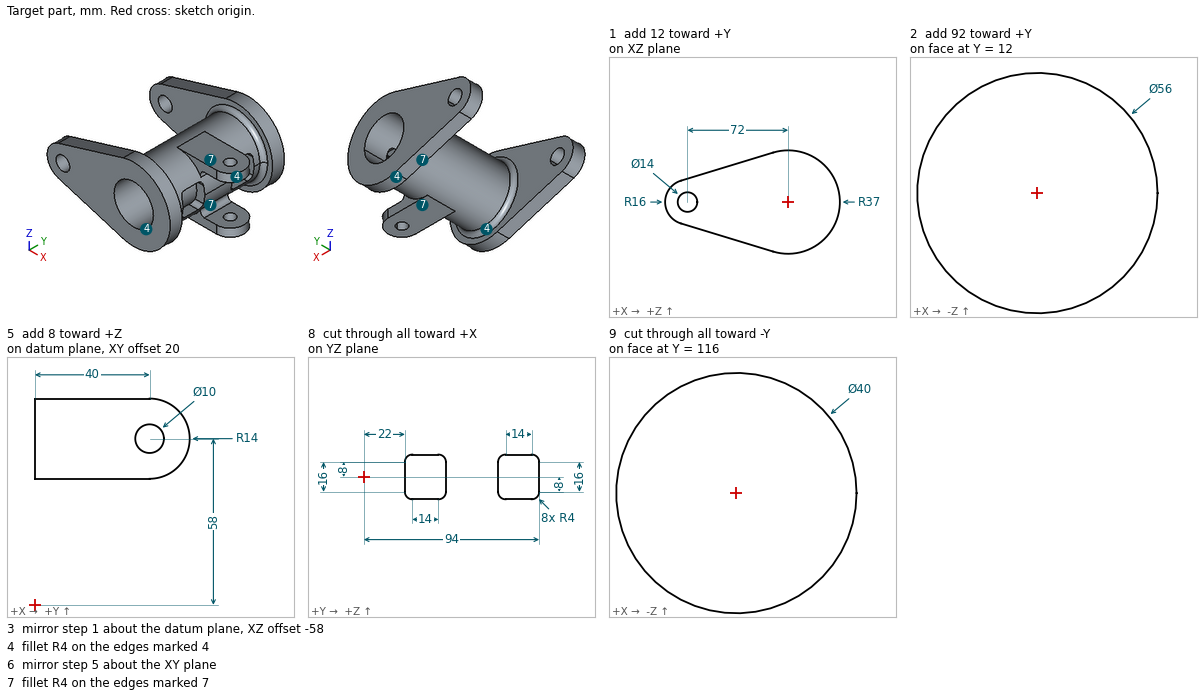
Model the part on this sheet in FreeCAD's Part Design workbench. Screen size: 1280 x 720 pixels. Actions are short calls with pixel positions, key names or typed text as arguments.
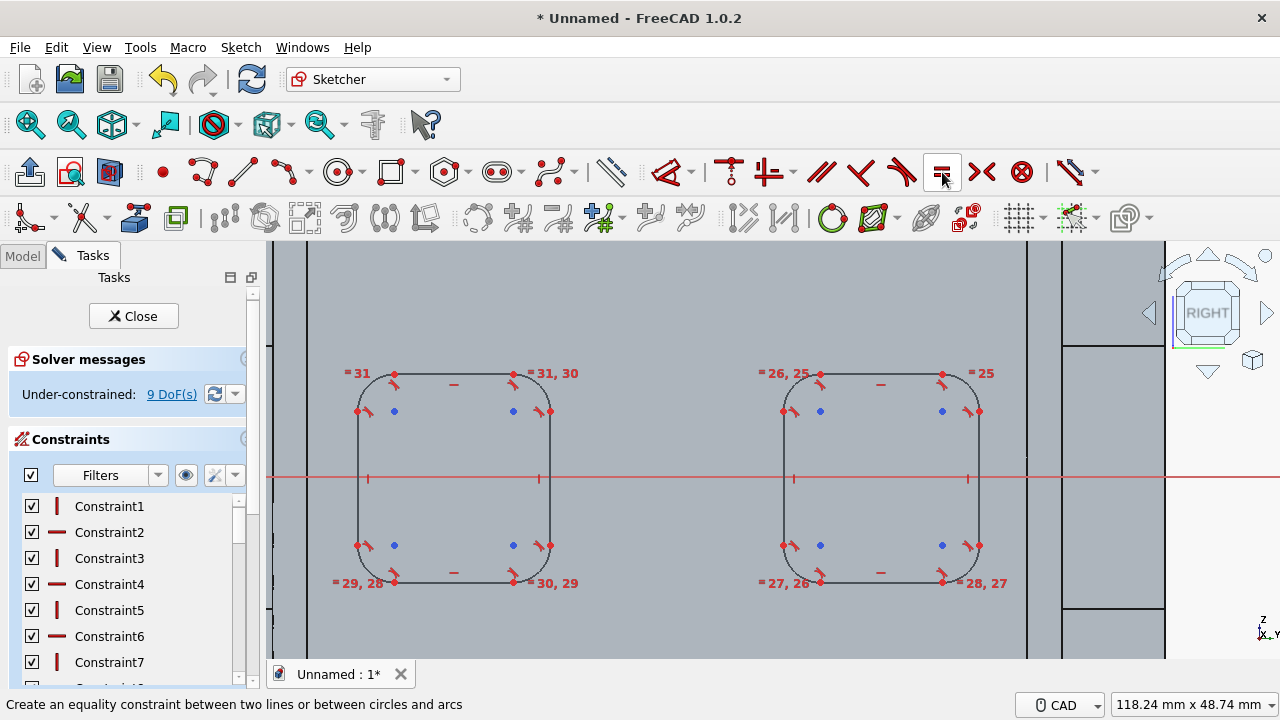
click(666, 172)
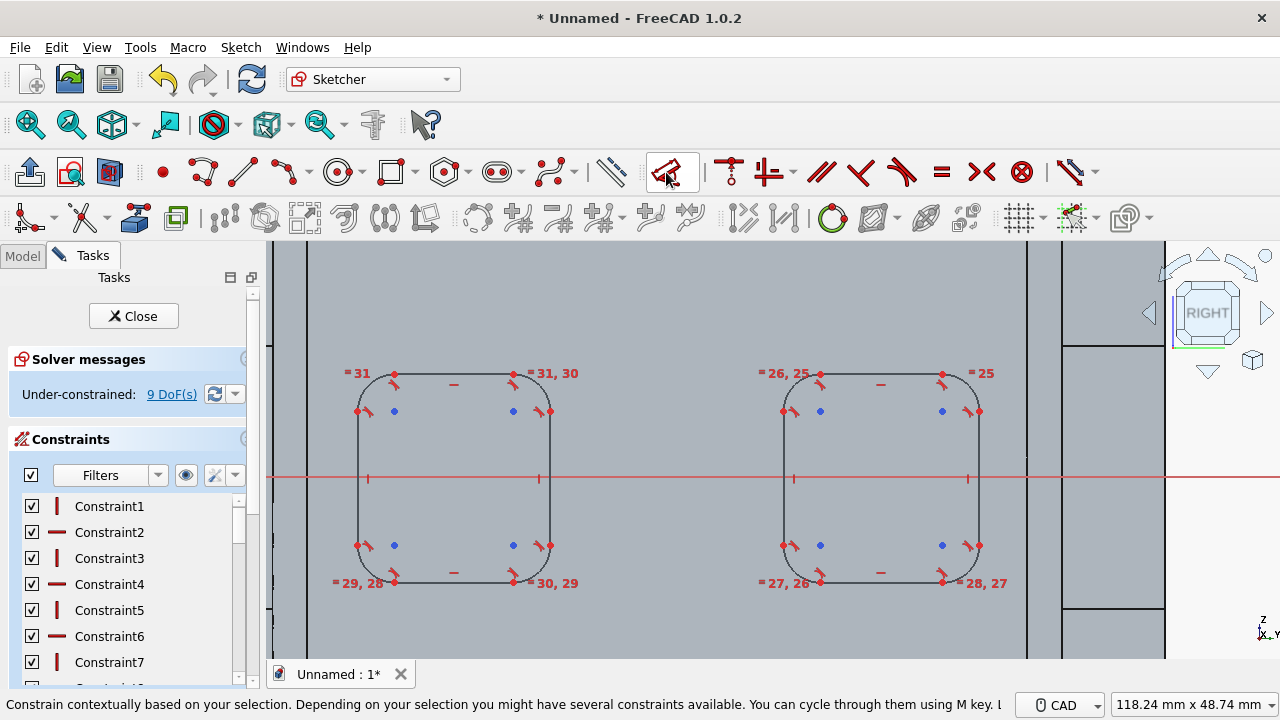
click(975, 395)
click(1004, 381)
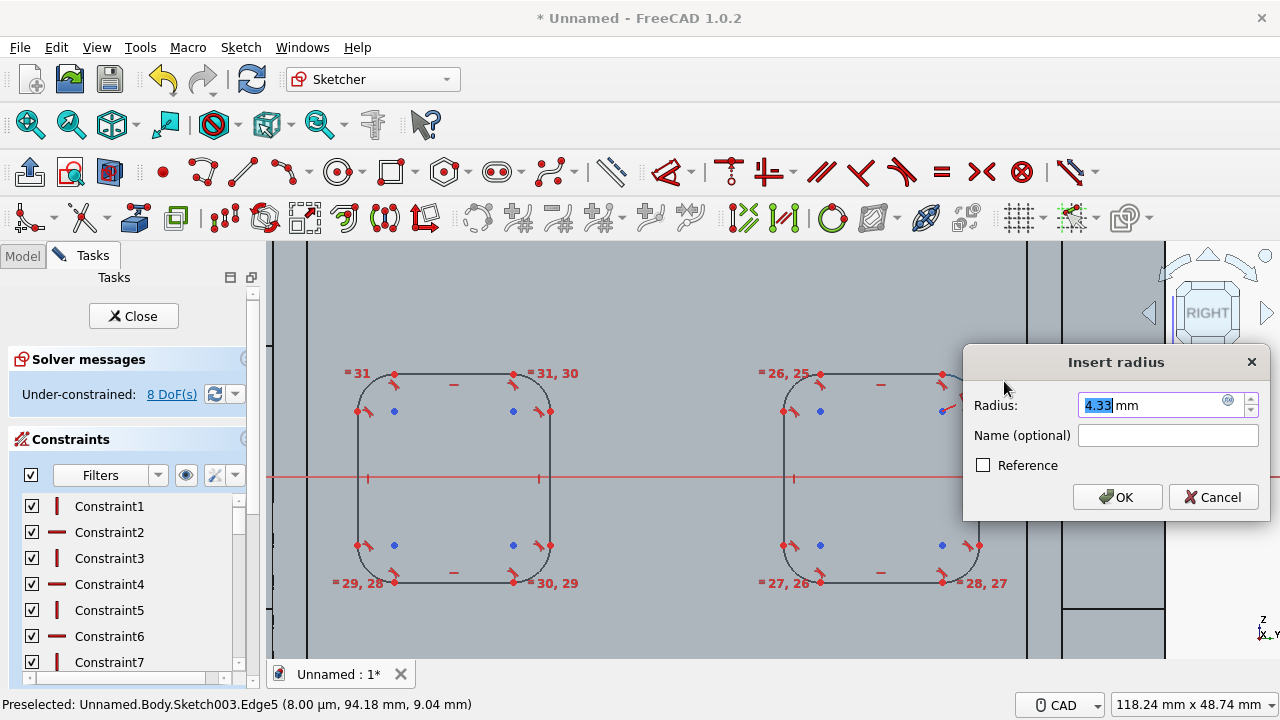
text(4)
key(Return)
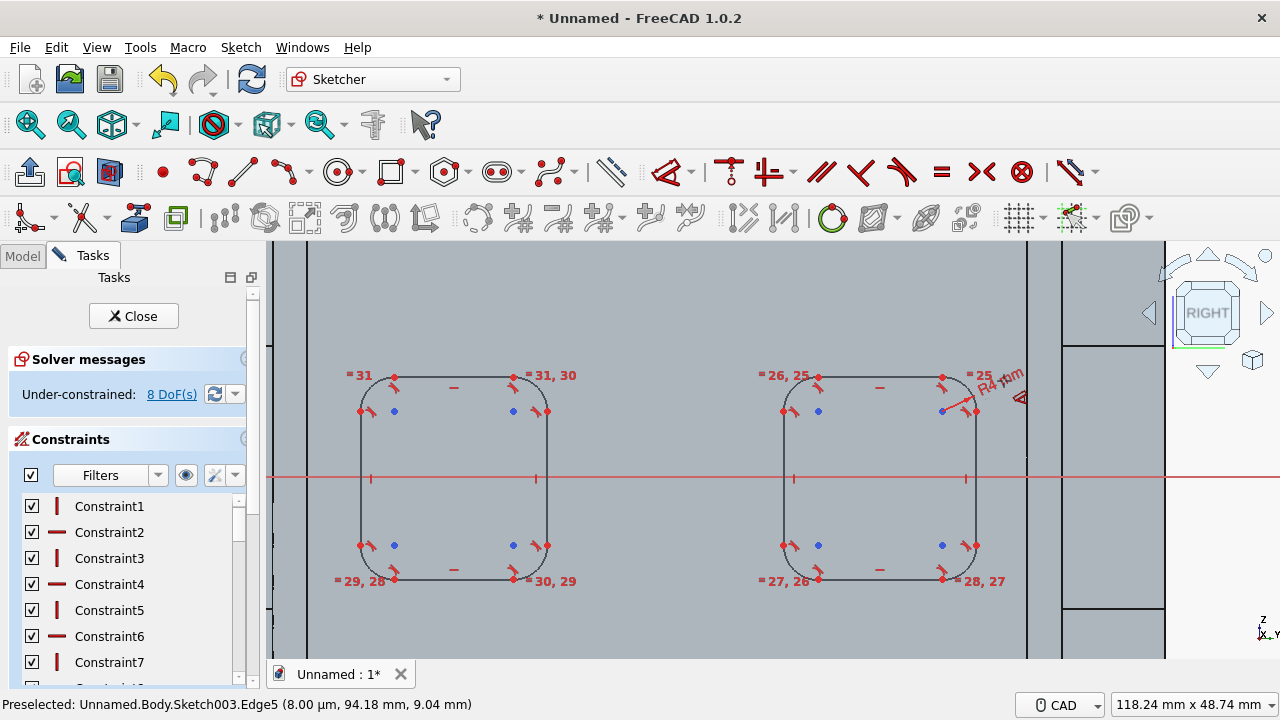
click(976, 505)
click(1010, 448)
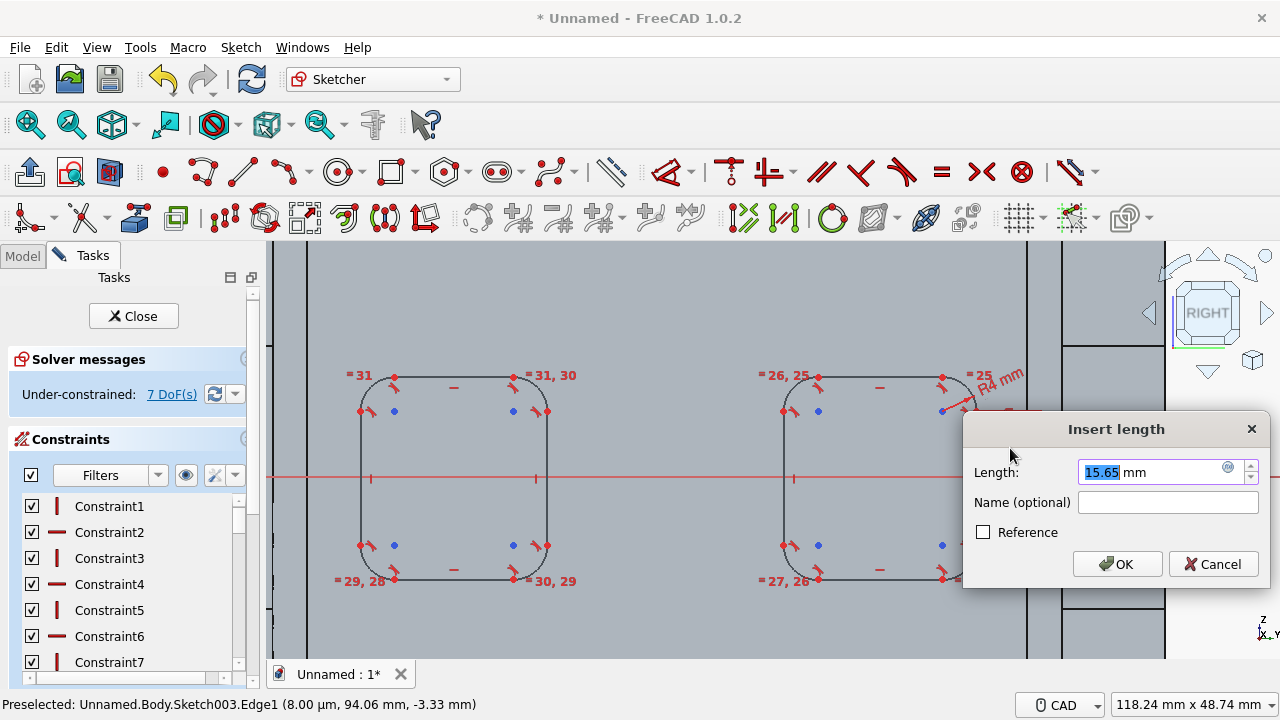
text(16)
key(Return)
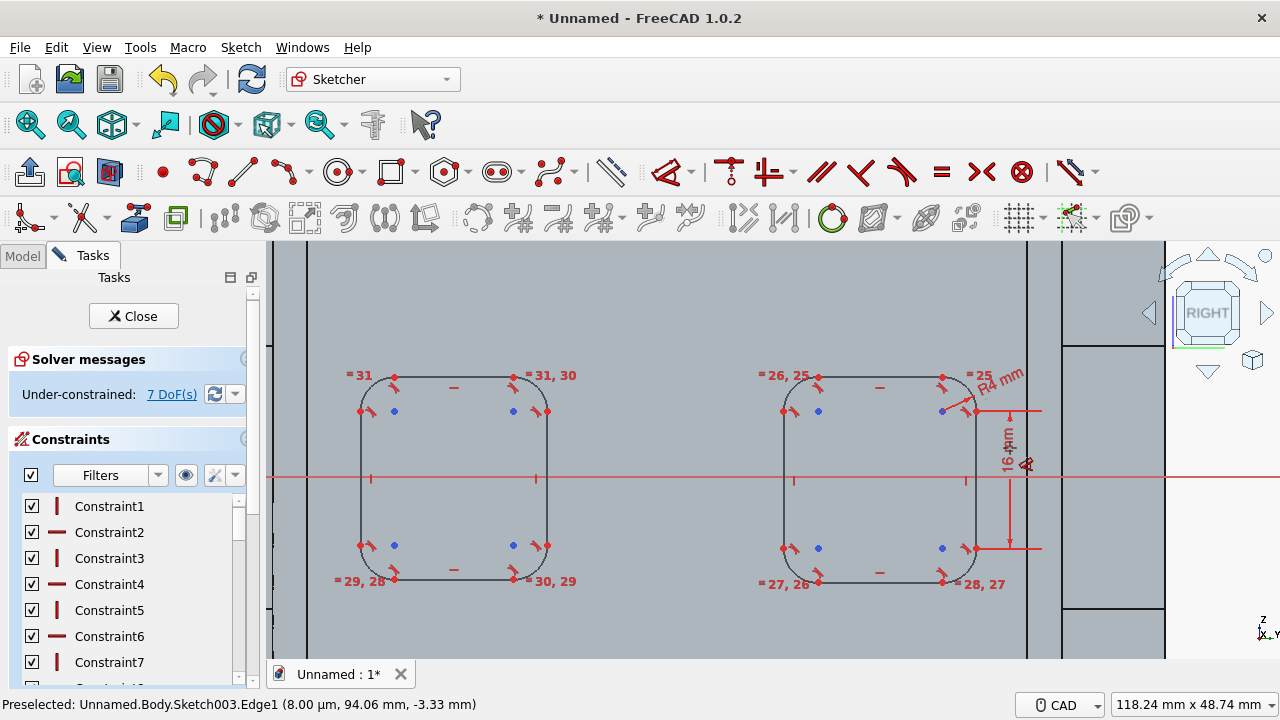
click(905, 377)
click(880, 343)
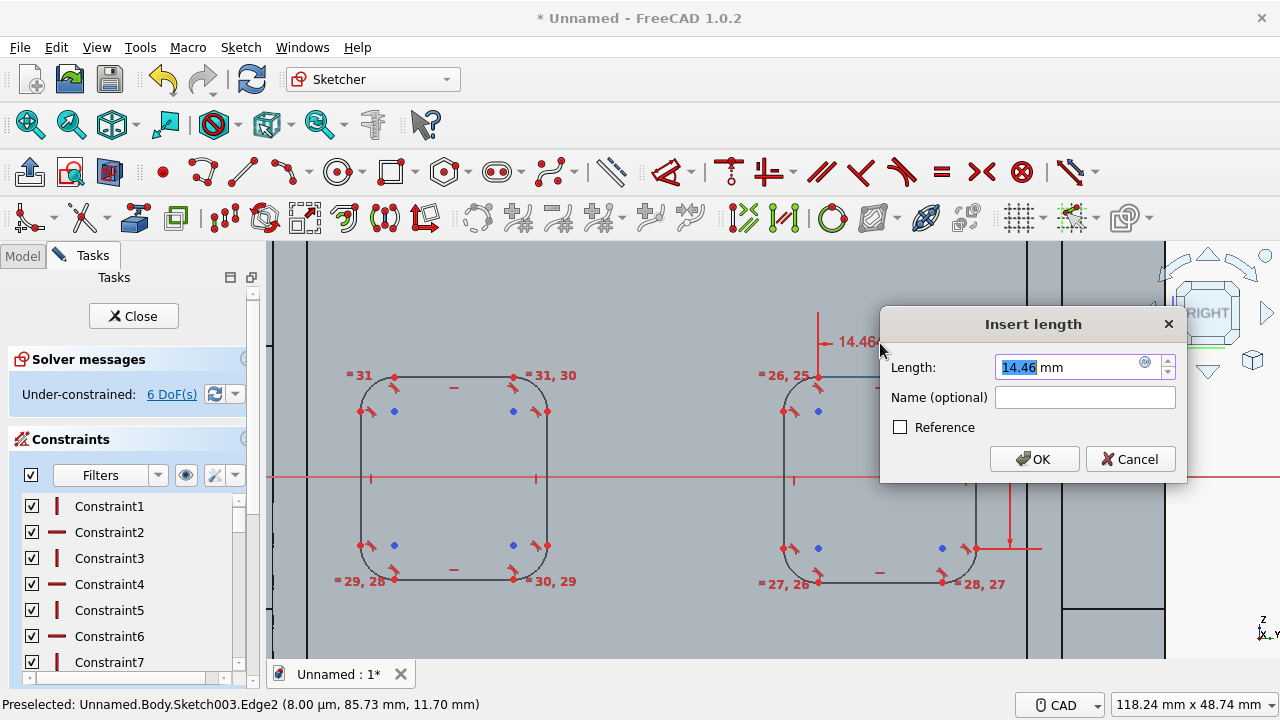
text(14)
key(Return)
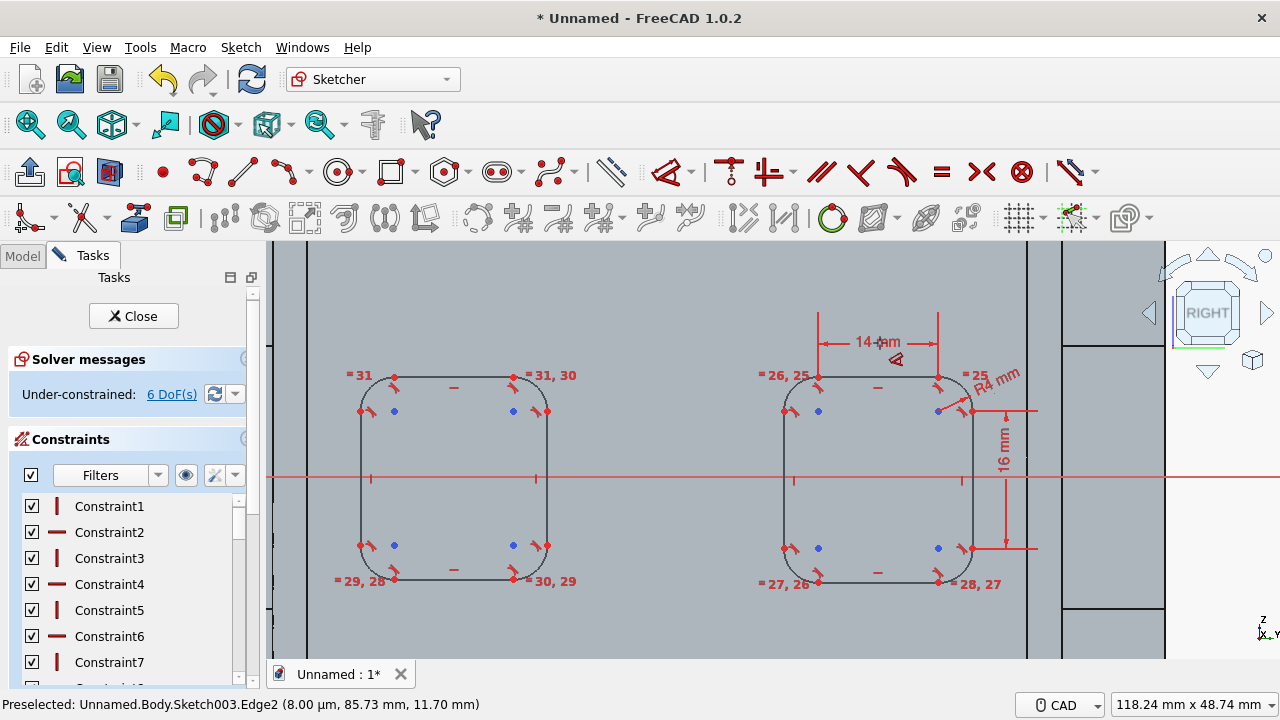
click(361, 452)
click(327, 448)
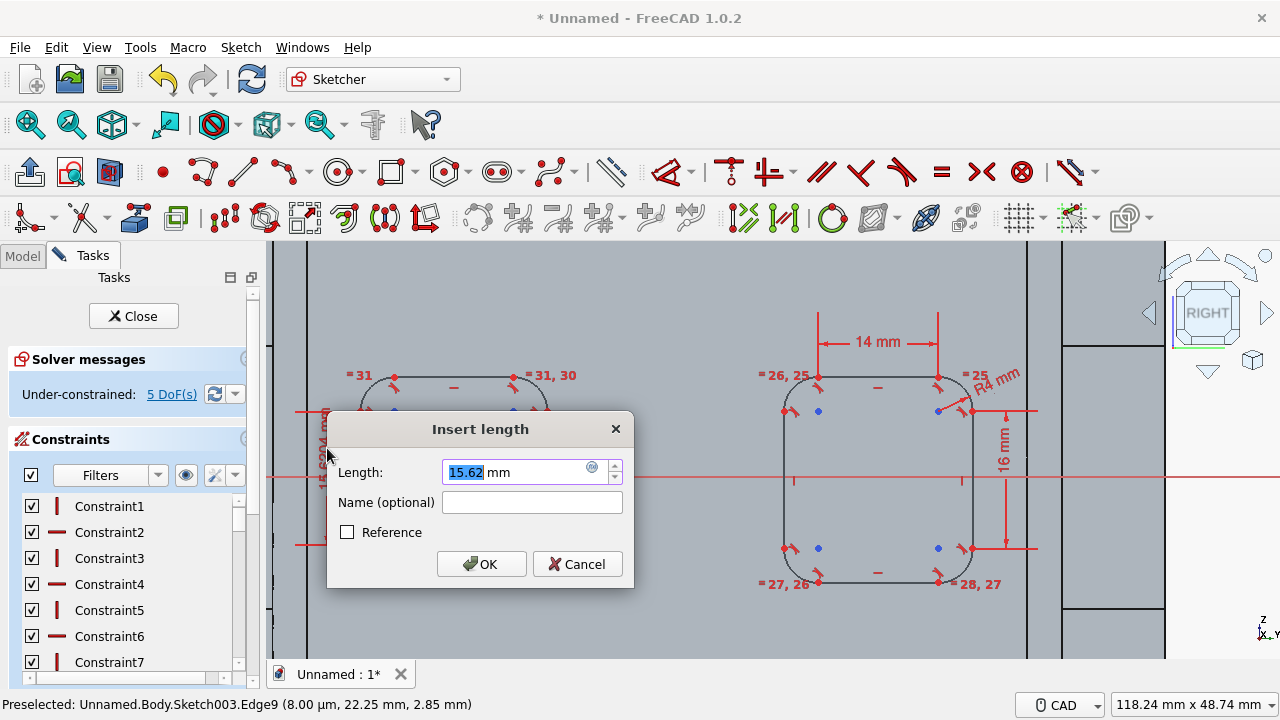
text(16)
key(Return)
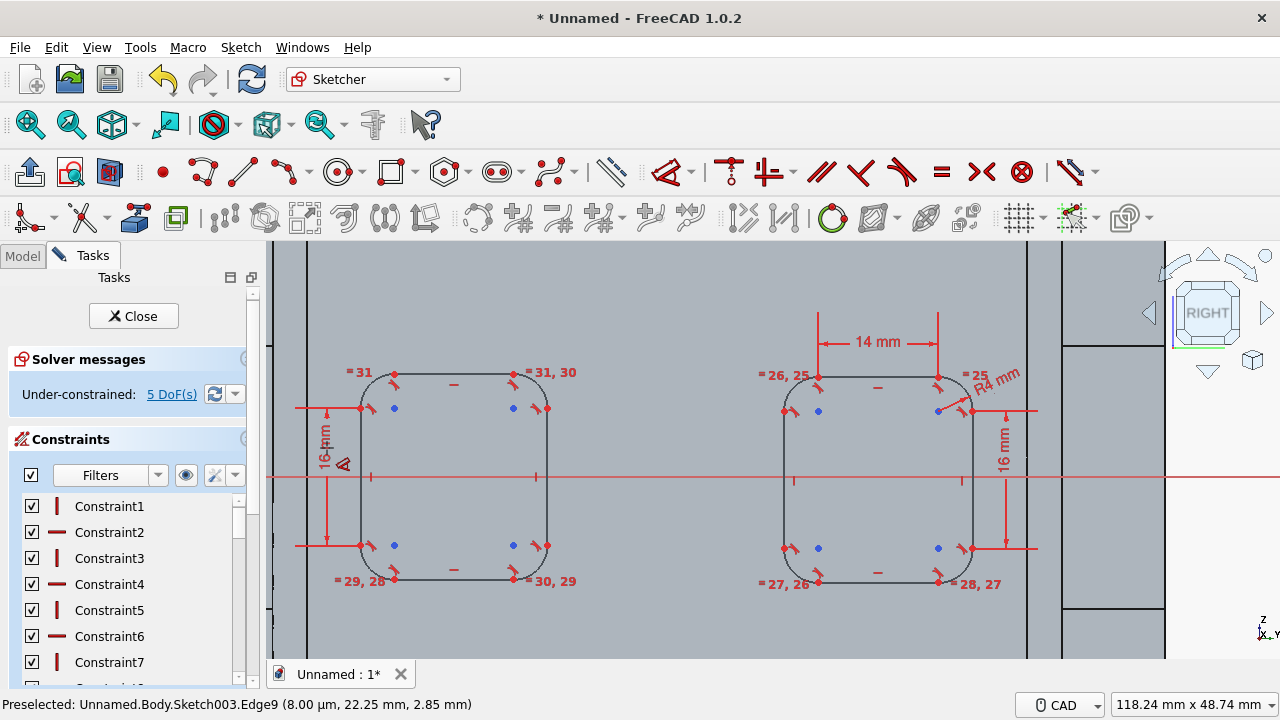
click(430, 580)
click(454, 614)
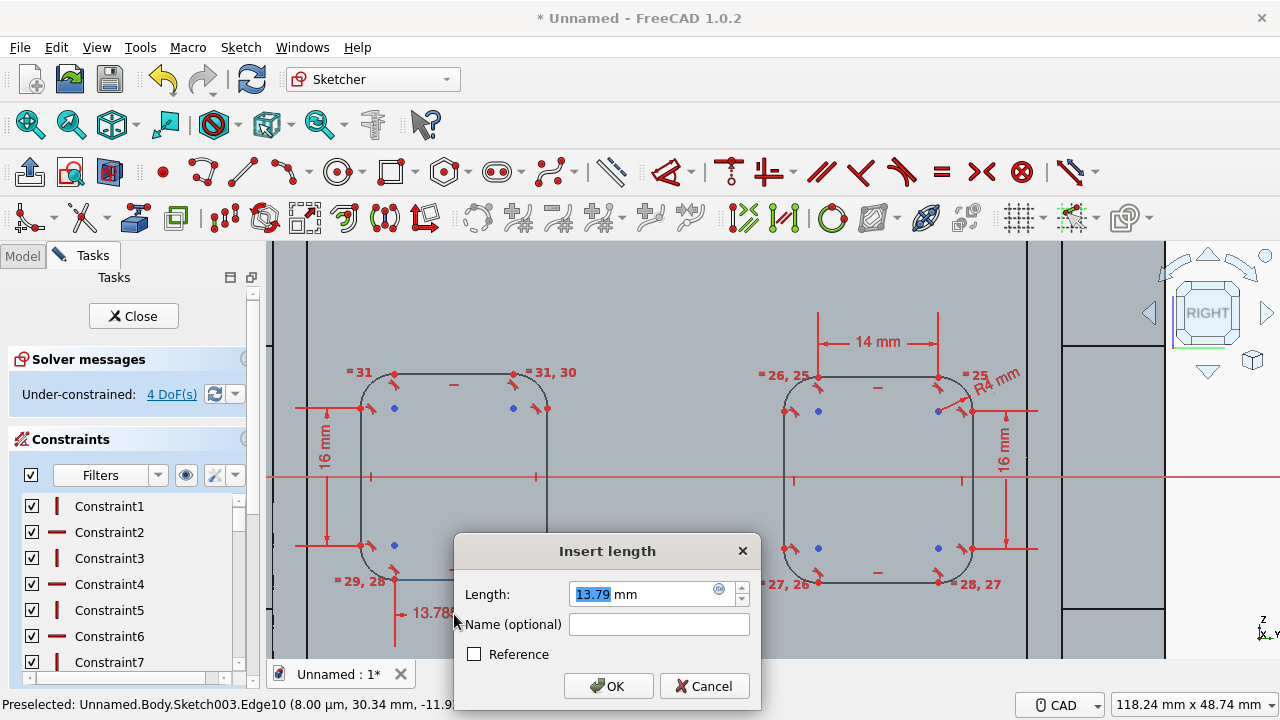
text(14)
key(Return)